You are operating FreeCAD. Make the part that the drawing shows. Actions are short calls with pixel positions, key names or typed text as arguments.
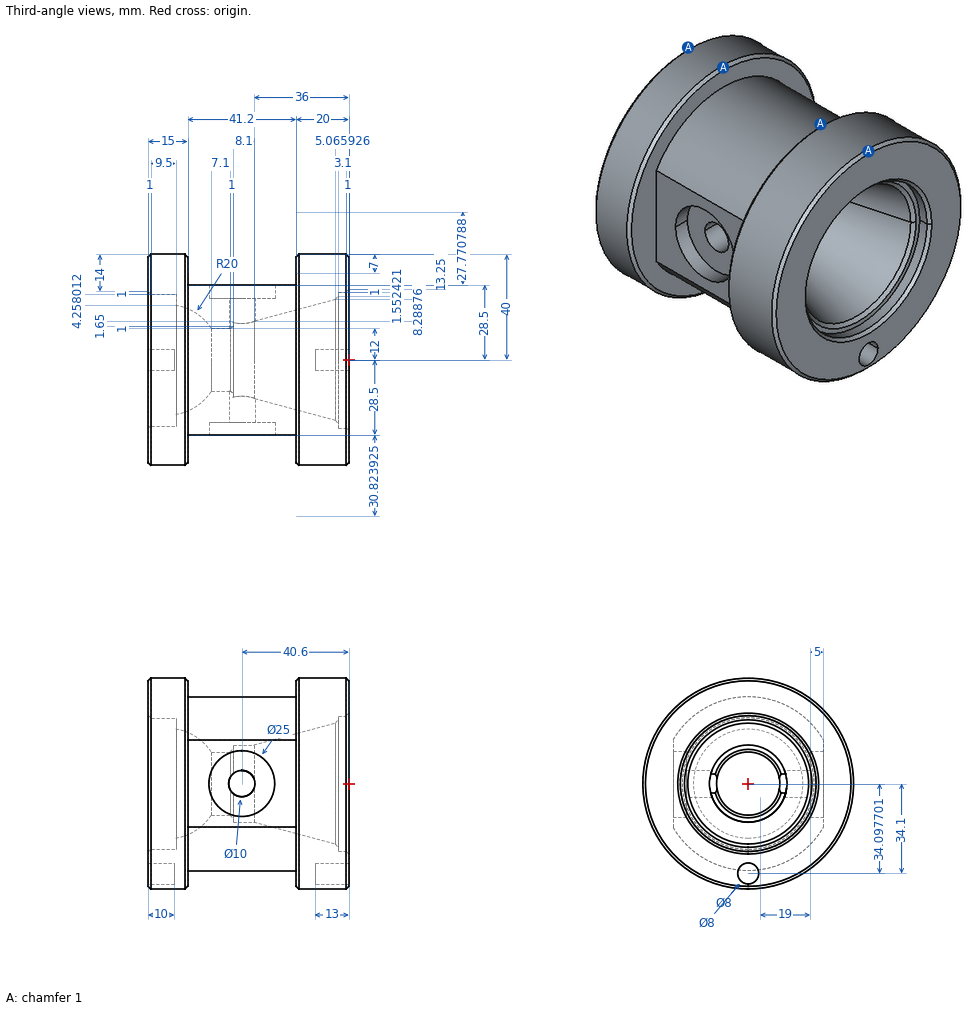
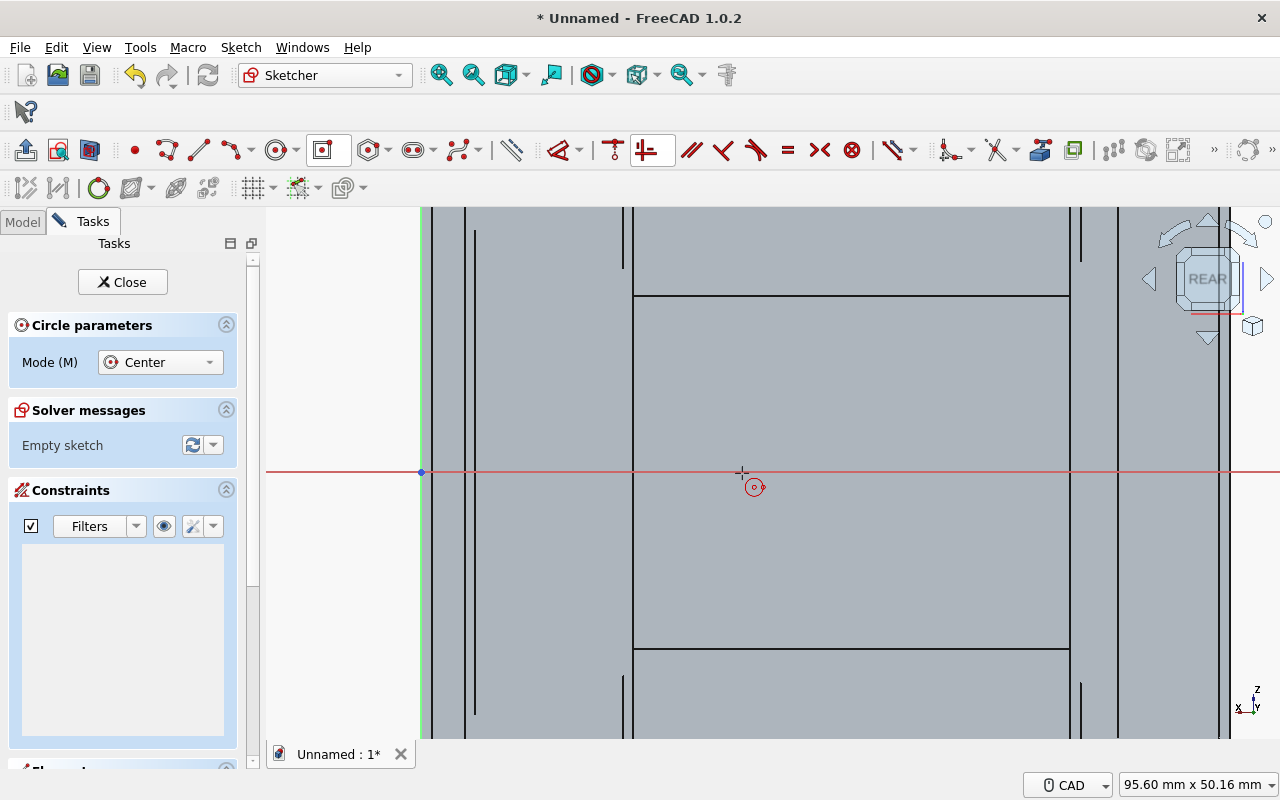
click(852, 472)
move(946, 378)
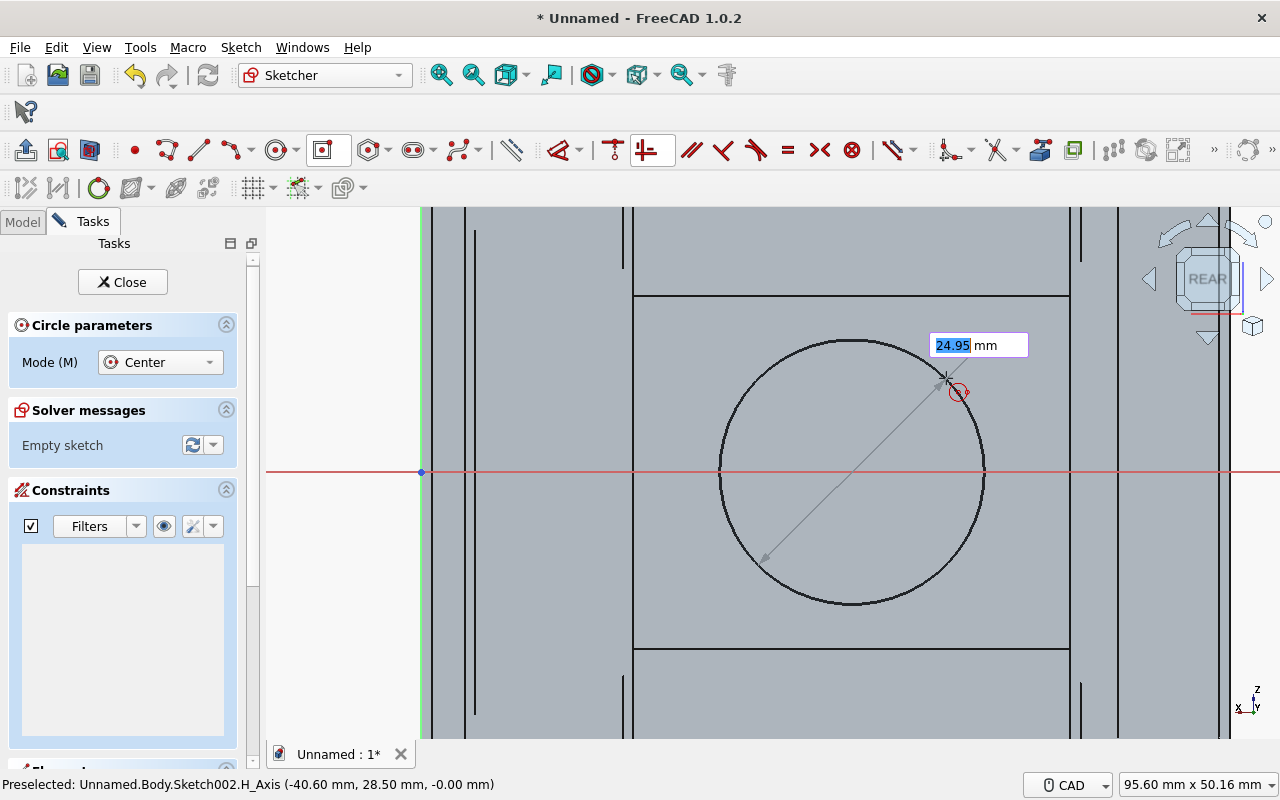
text(25)
key(Return)
key(Escape)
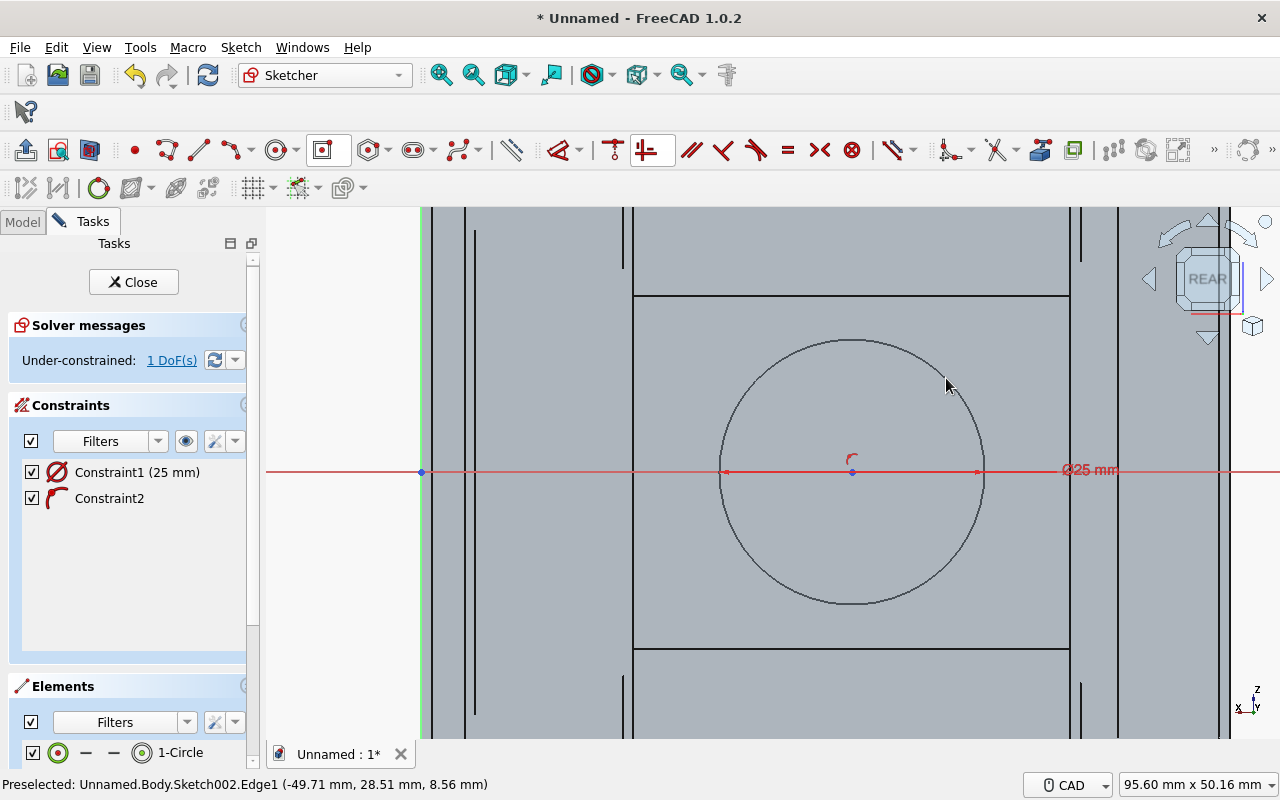
click(558, 150)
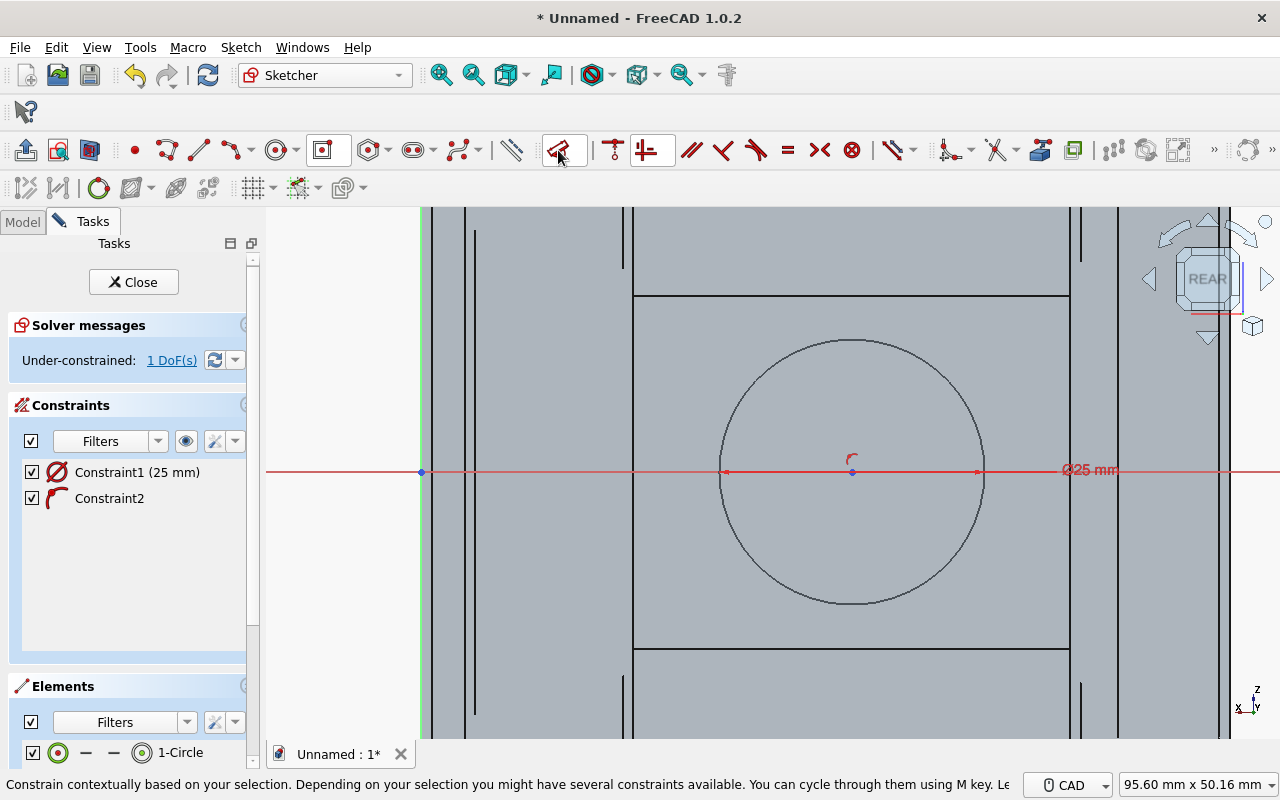
click(852, 472)
click(637, 506)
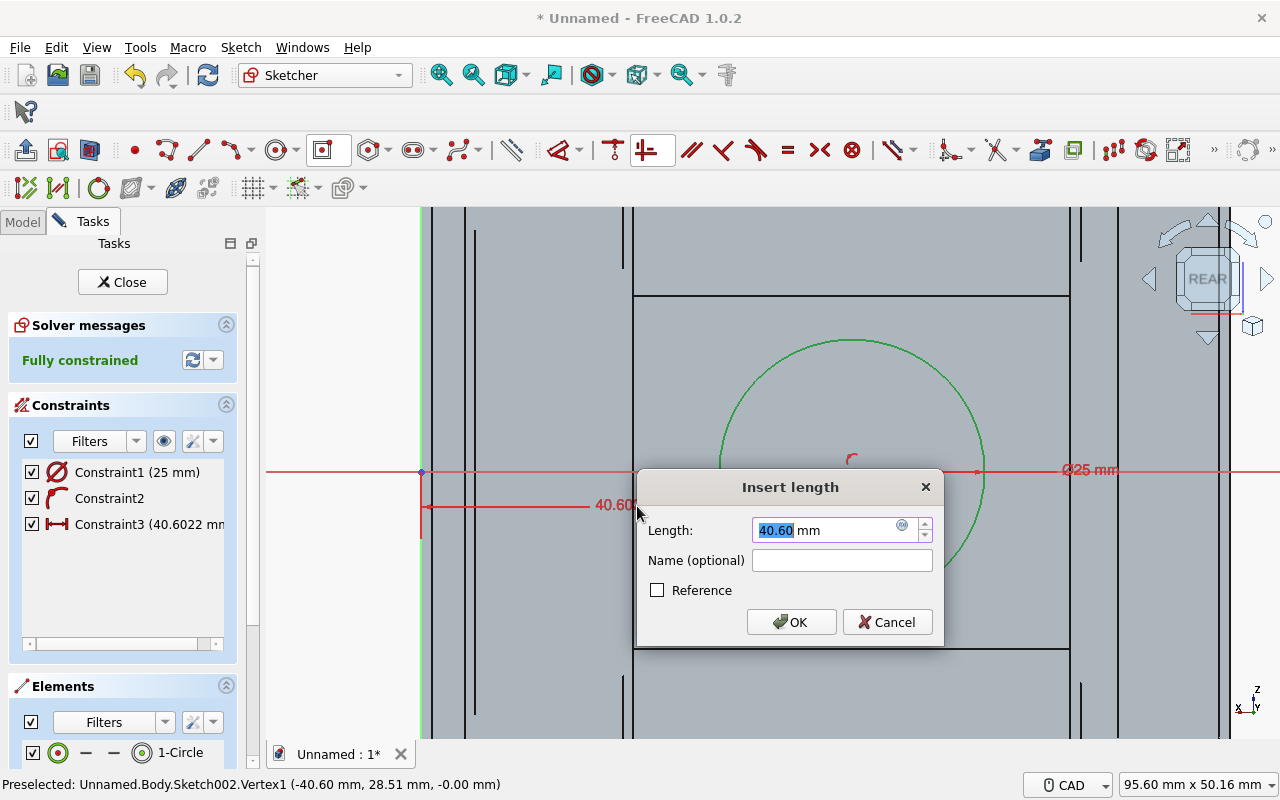
text(40.6)
key(Return)
key(Escape)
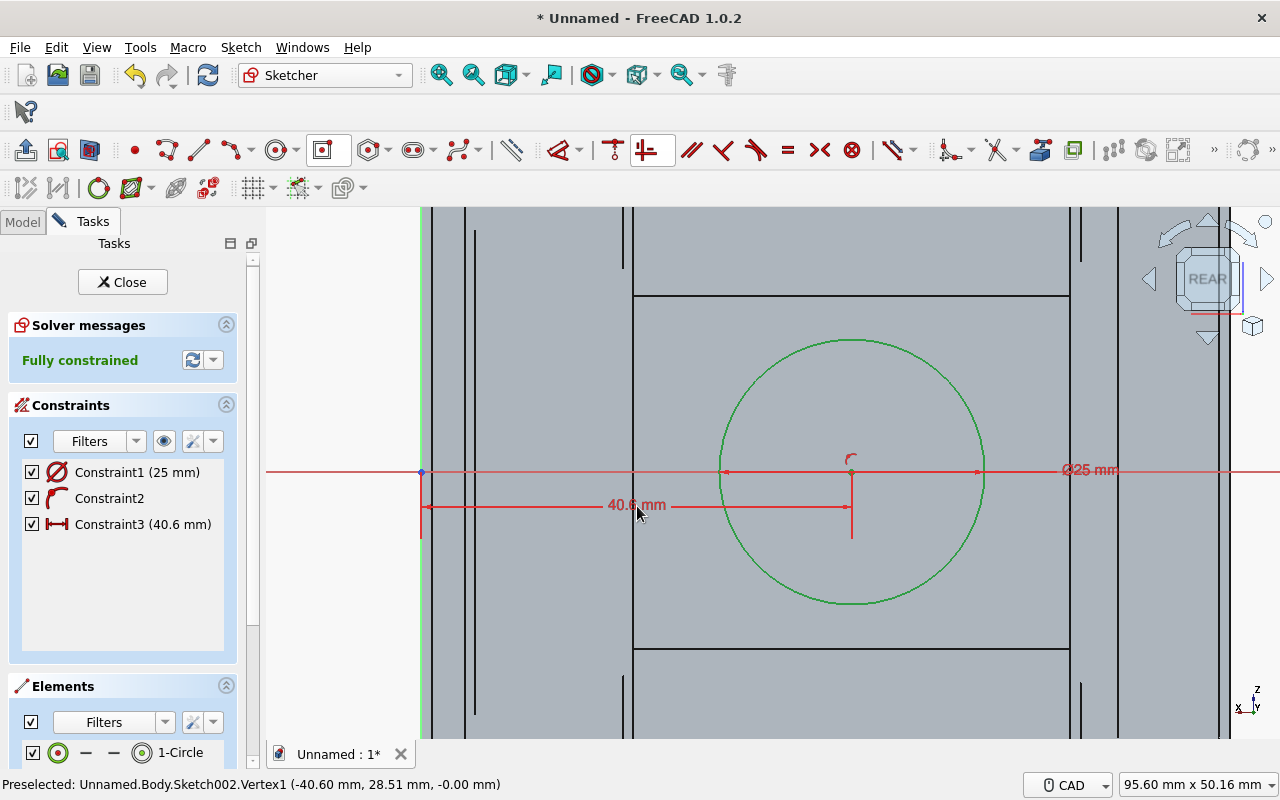
click(123, 282)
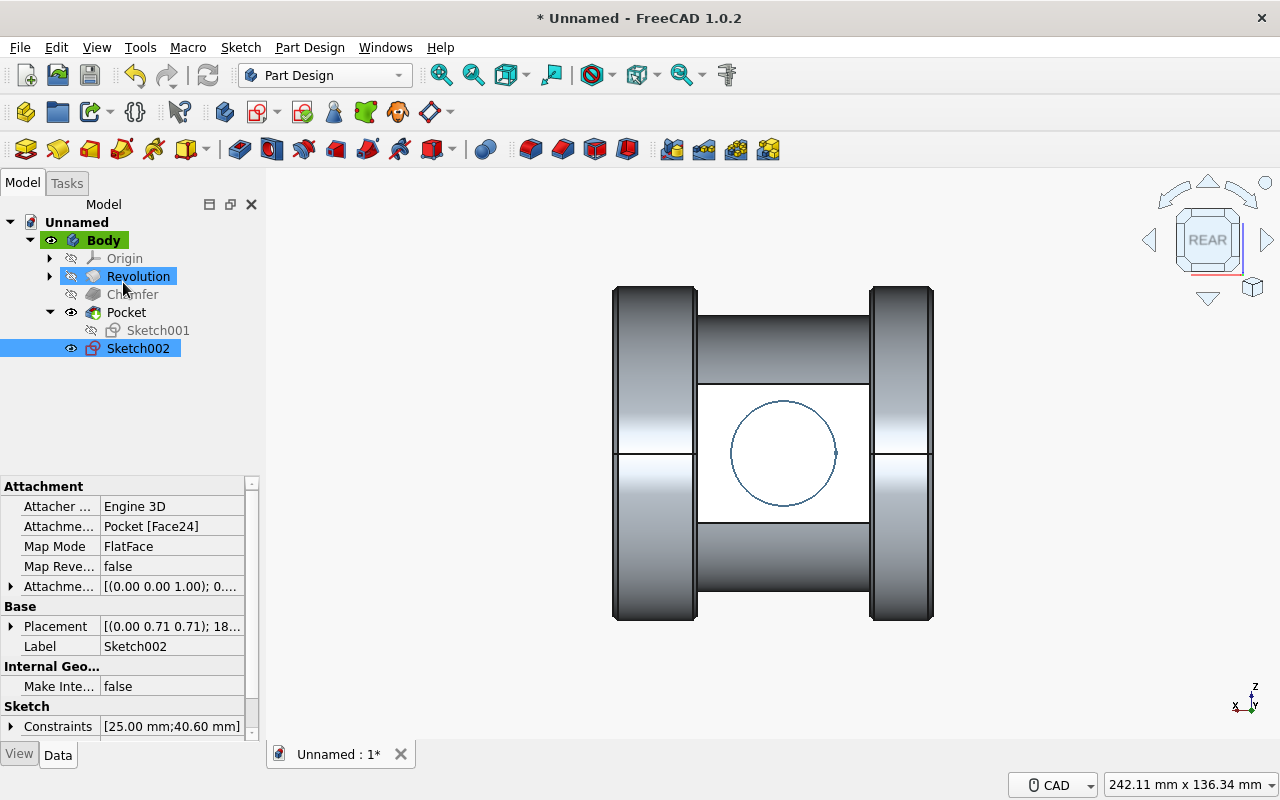
click(240, 150)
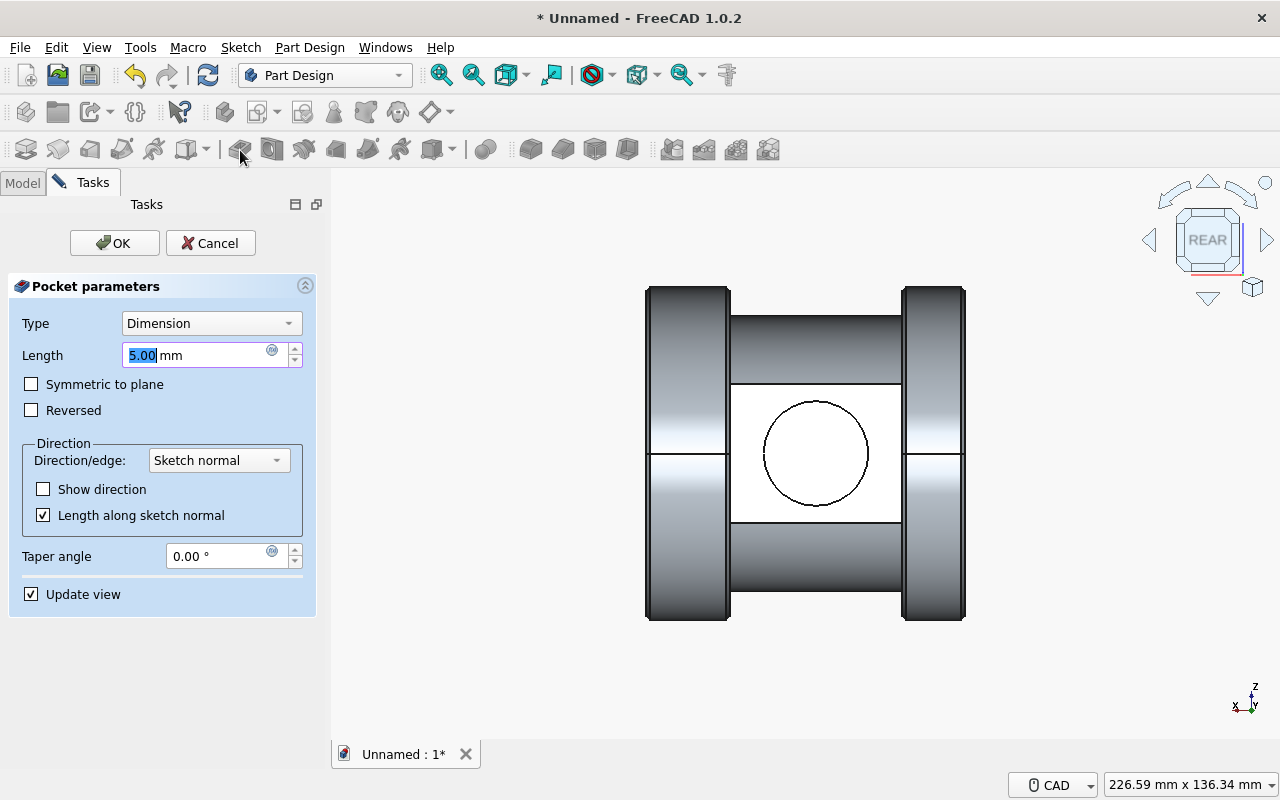
text(5)
key(Tab)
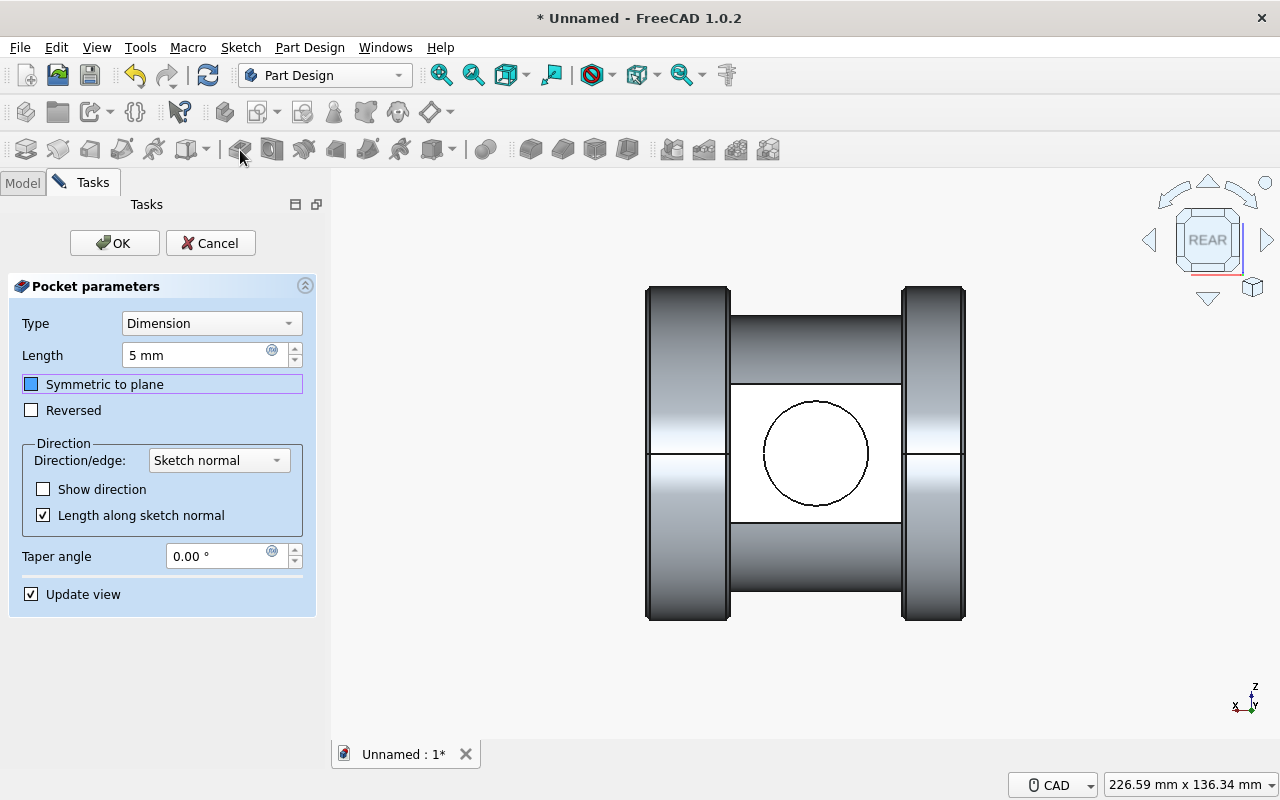
click(115, 243)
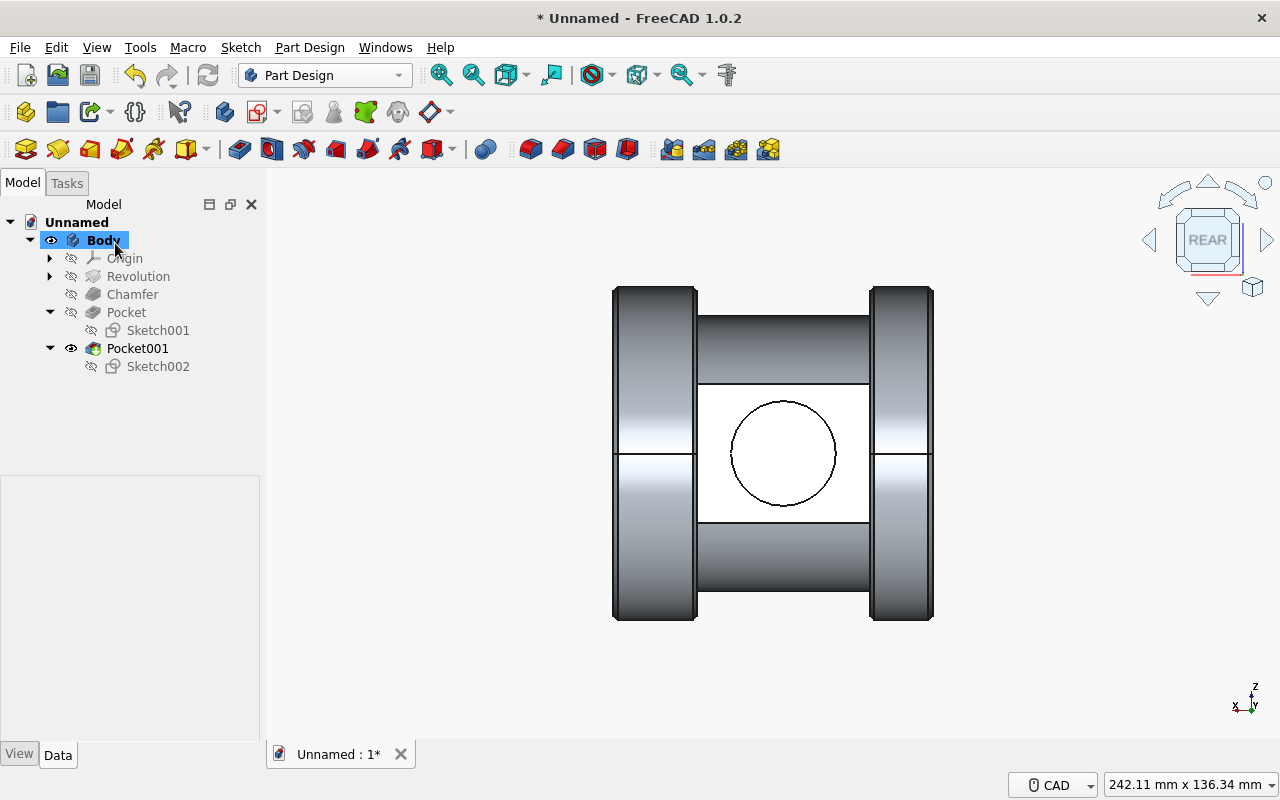
click(783, 452)